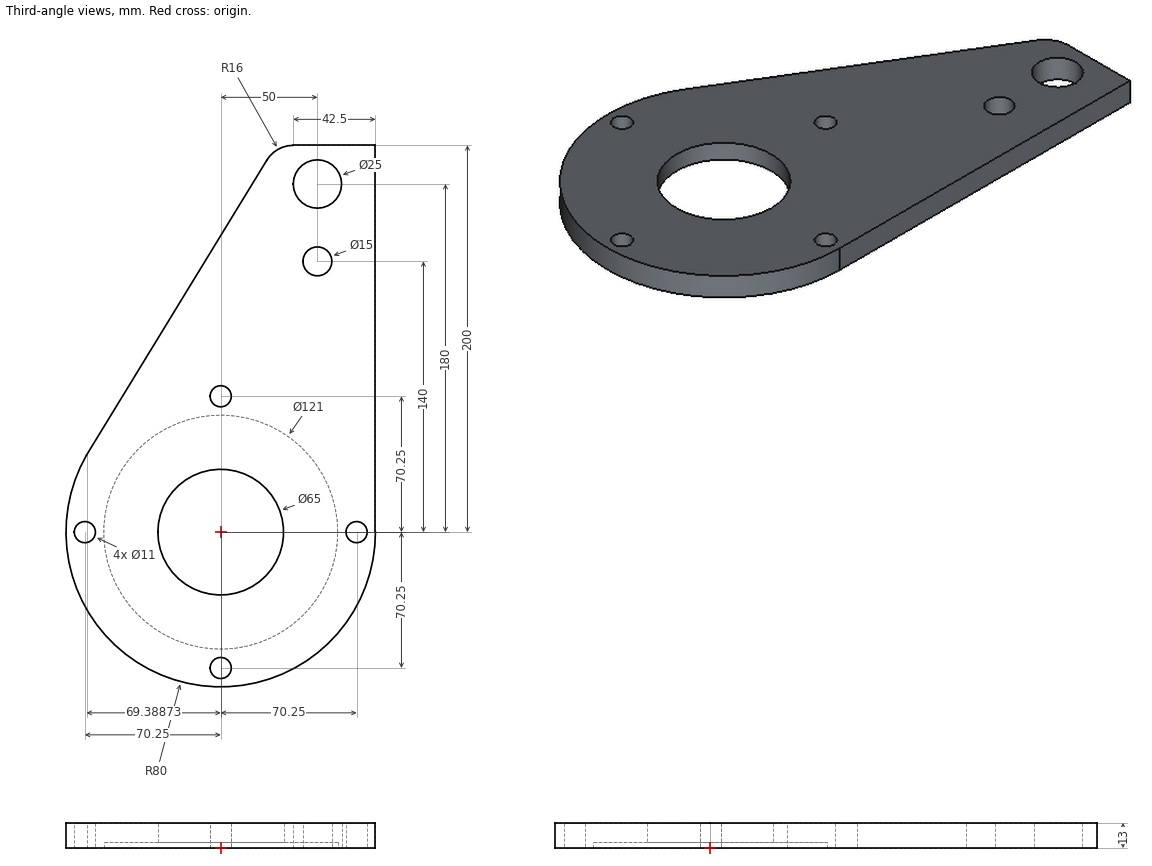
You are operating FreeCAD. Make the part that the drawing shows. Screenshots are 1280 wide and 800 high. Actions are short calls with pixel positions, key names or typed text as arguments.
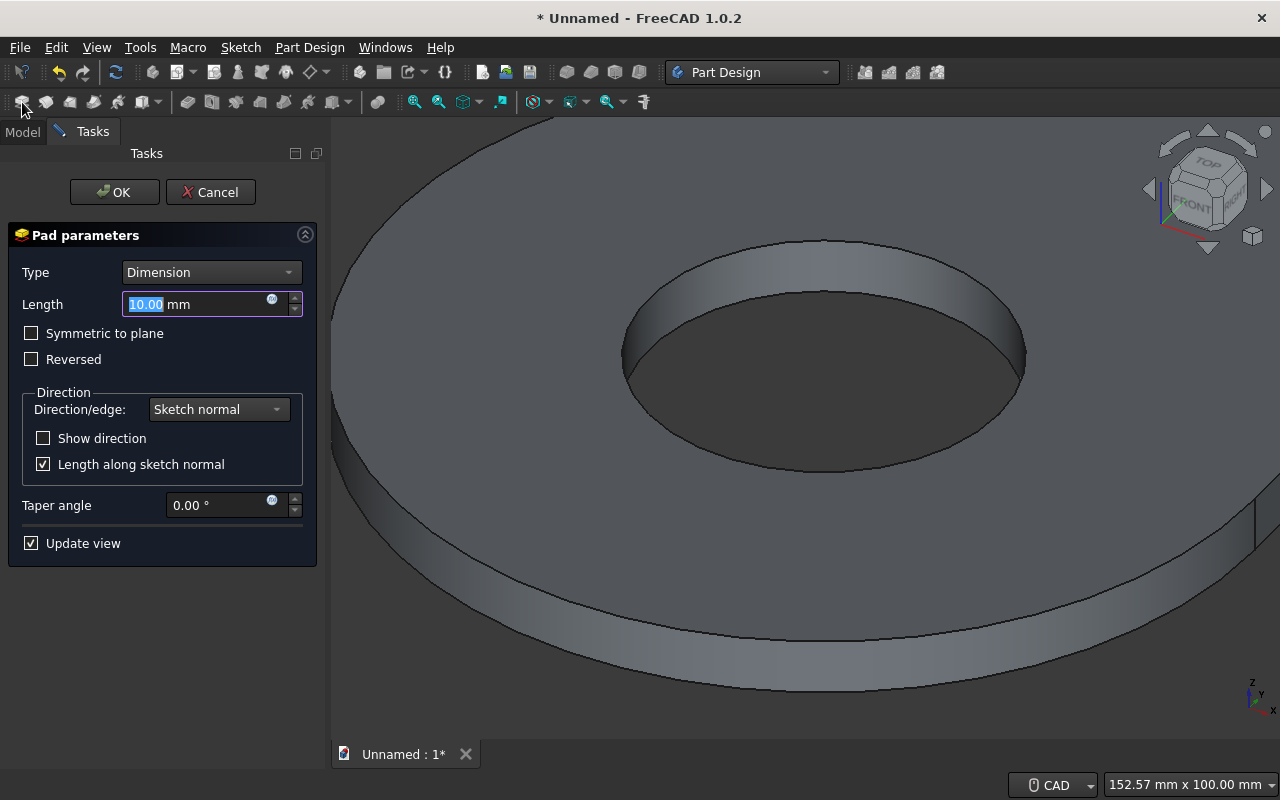
text(13)
key(Tab)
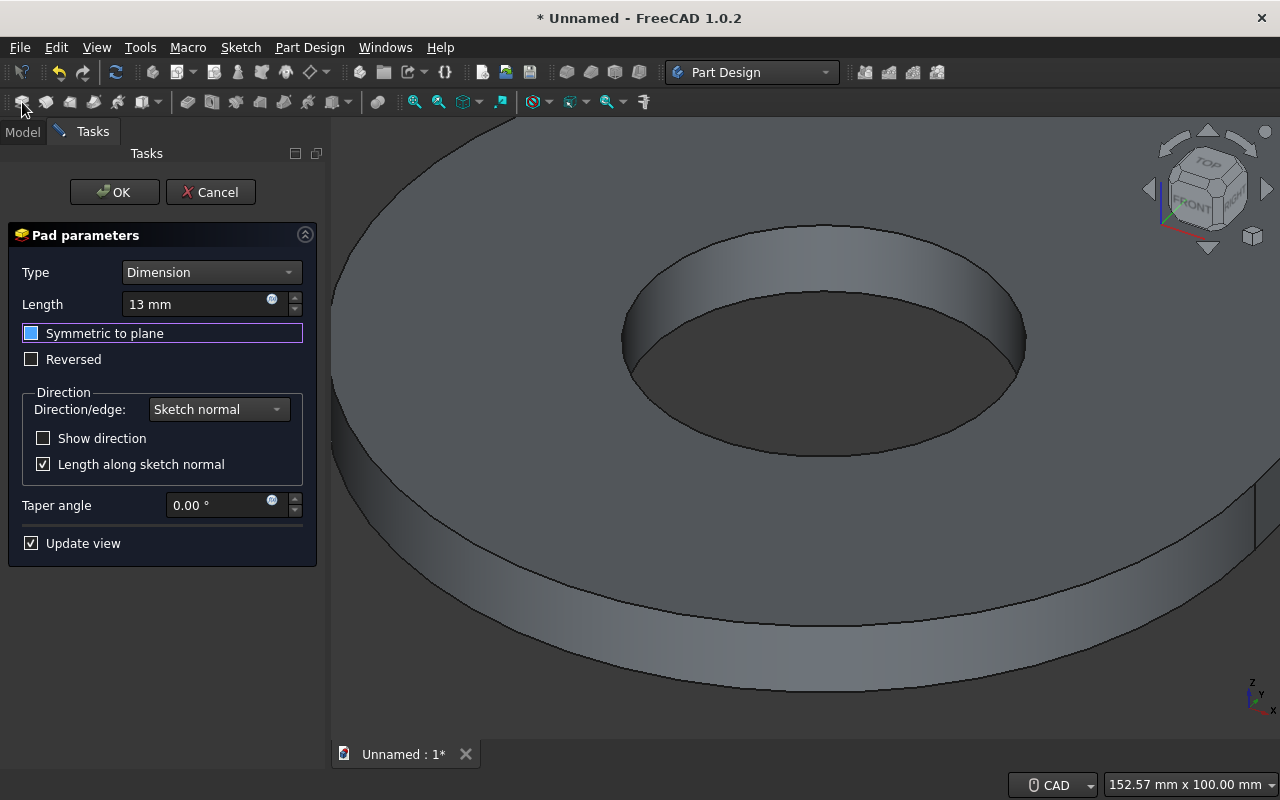
click(115, 192)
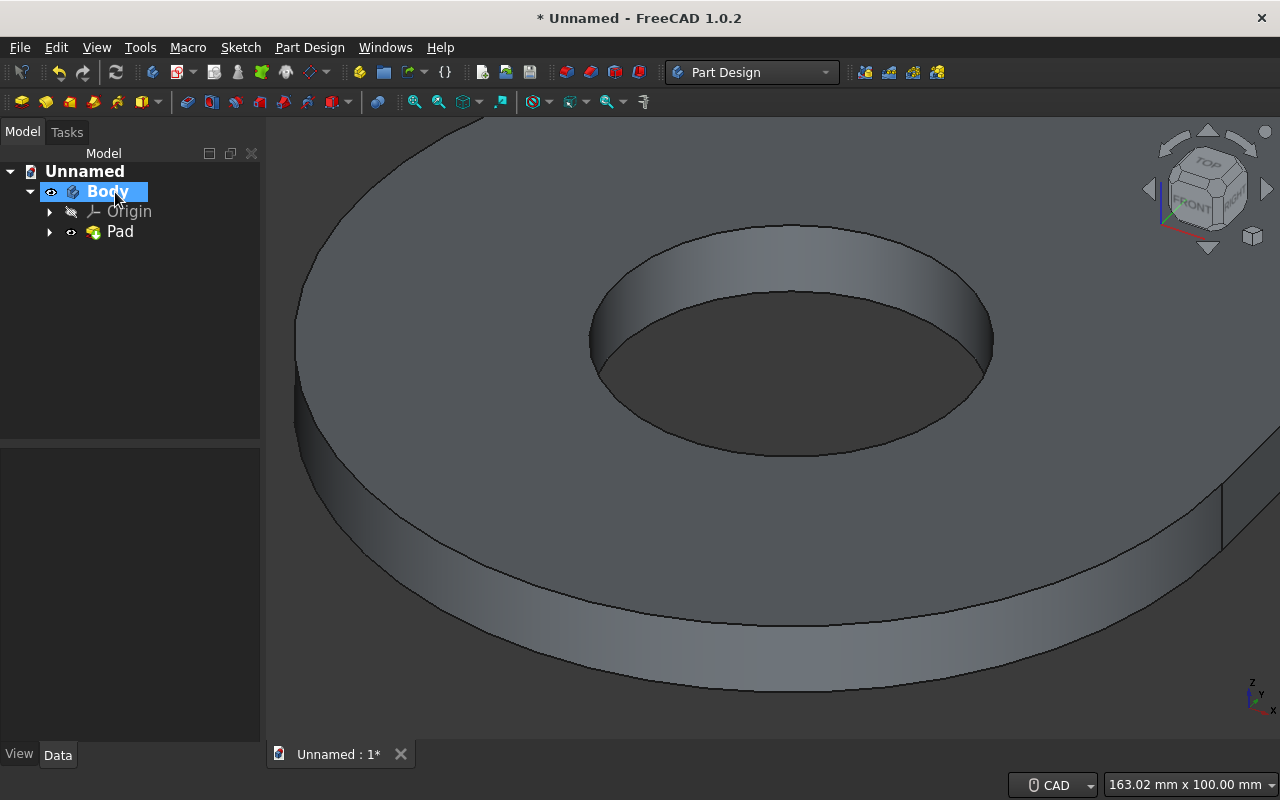
click(416, 102)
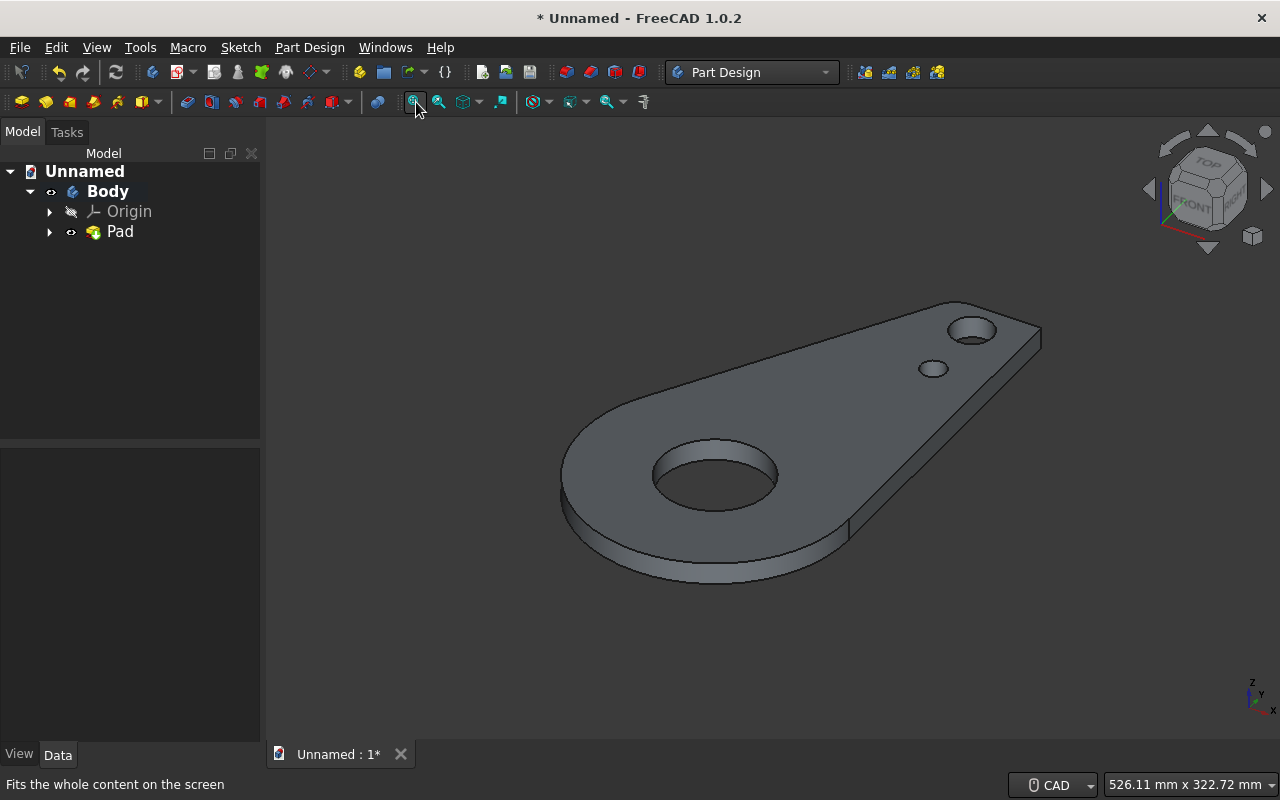
click(50, 212)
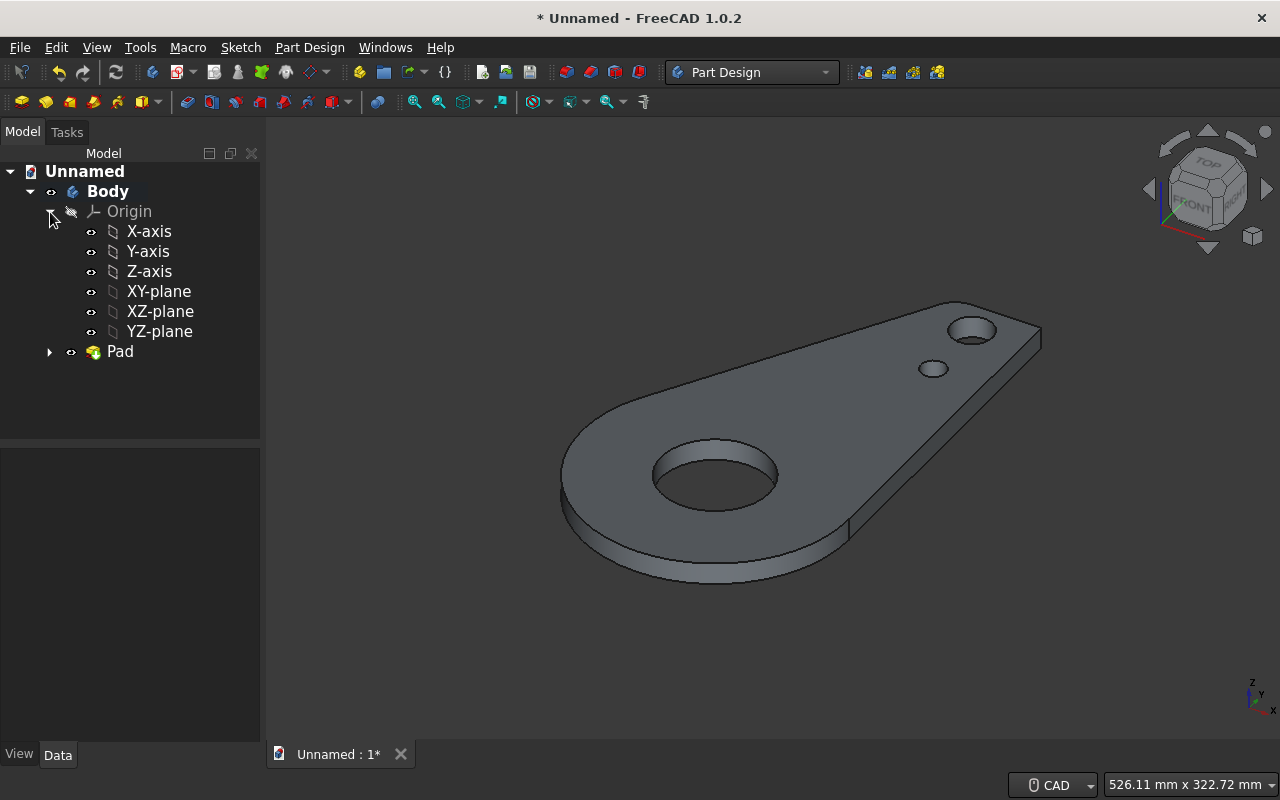
click(136, 292)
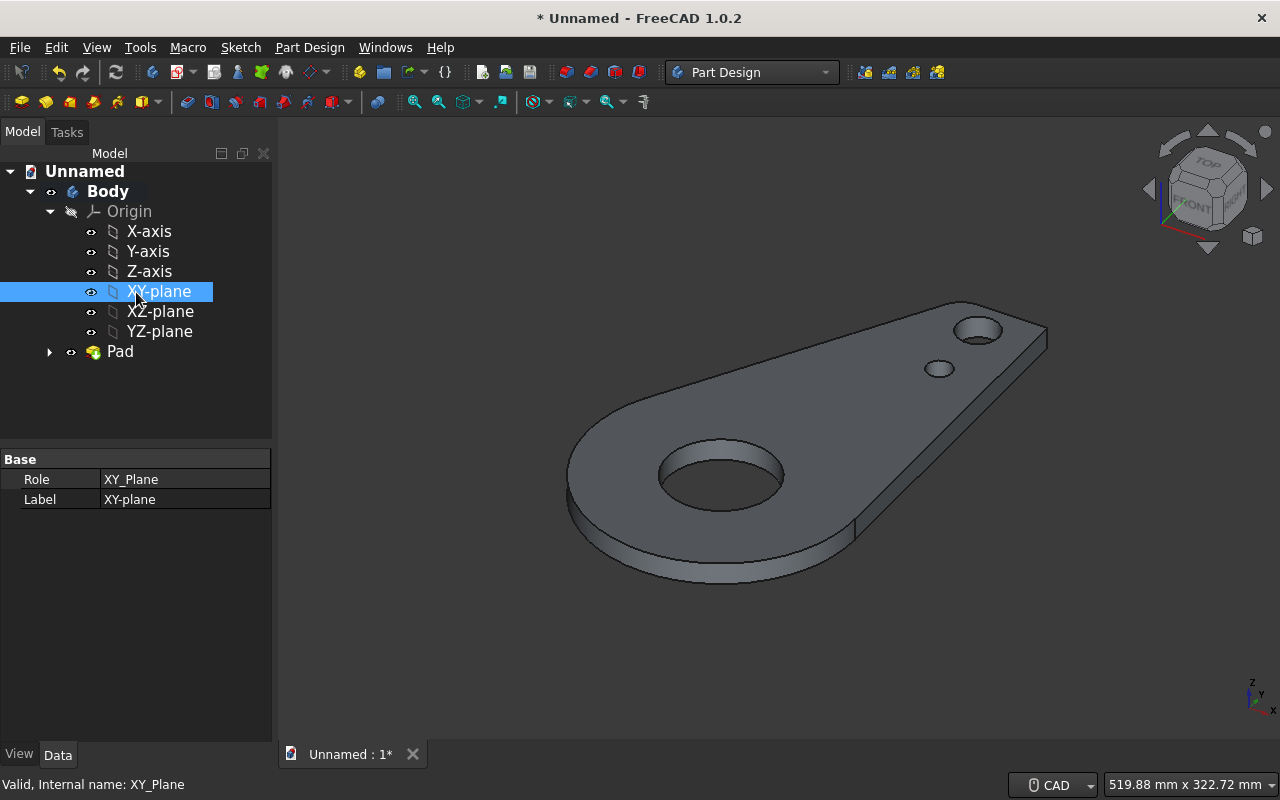
click(310, 72)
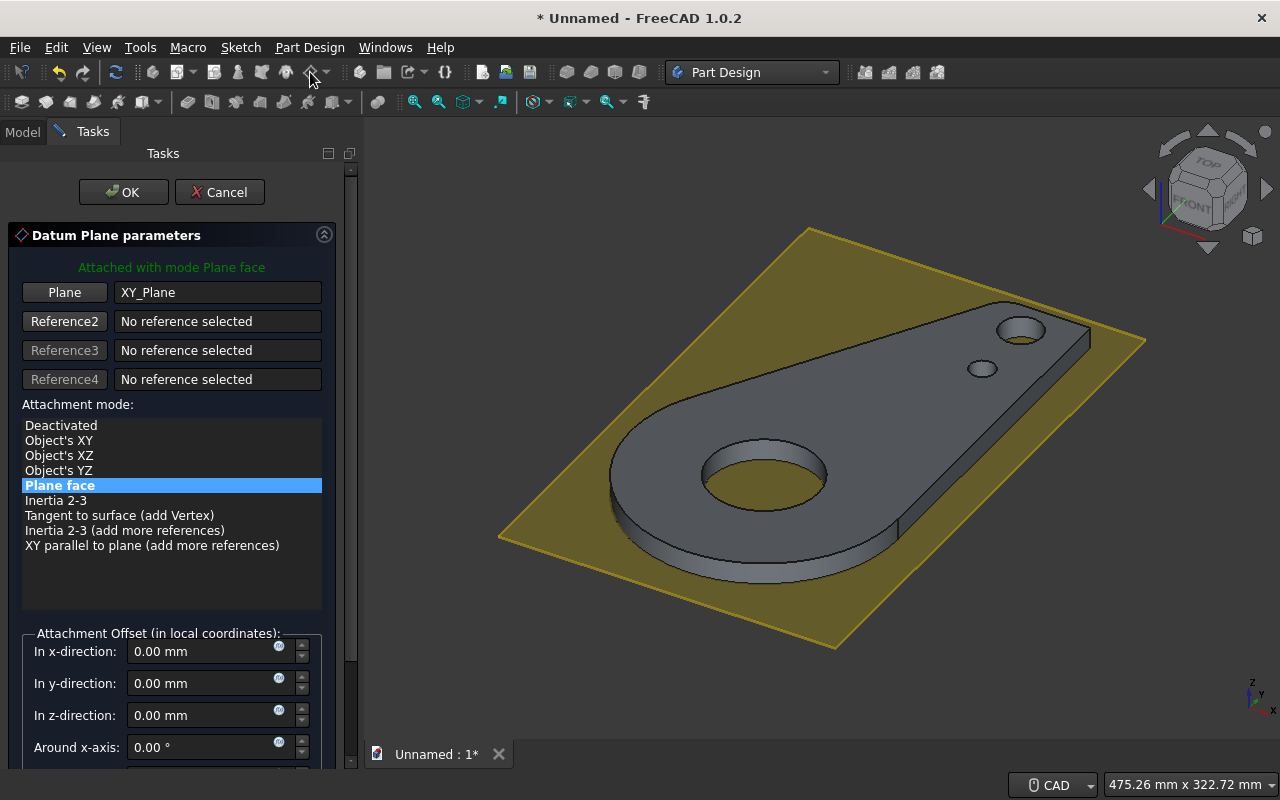
triple_click(210, 715)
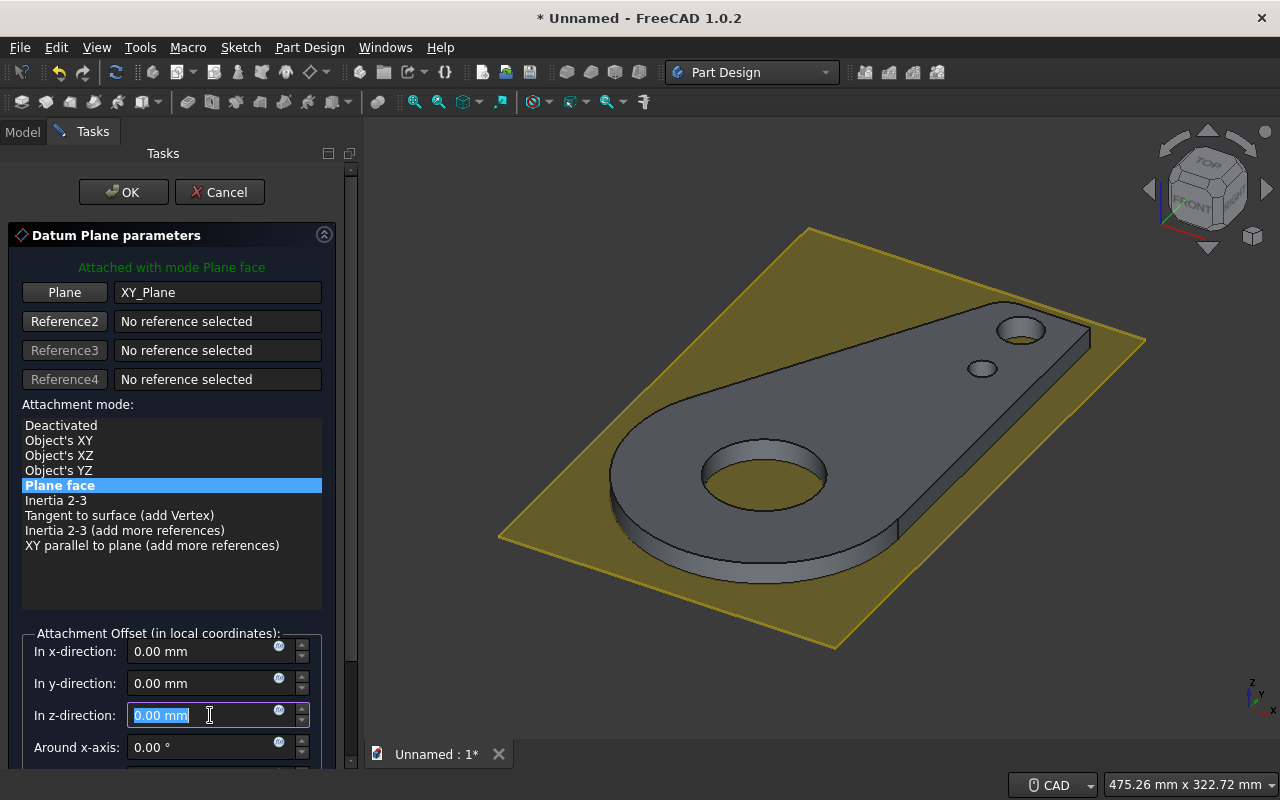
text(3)
key(Tab)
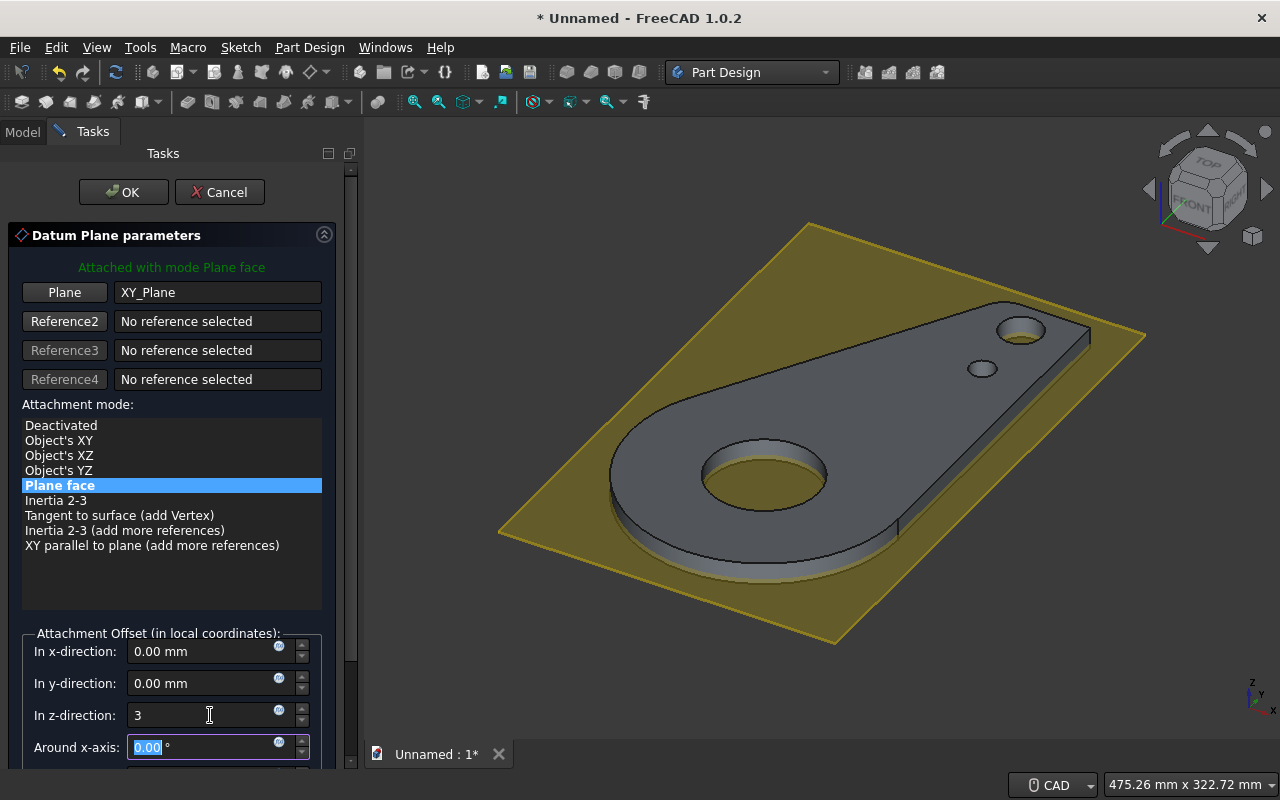
click(124, 192)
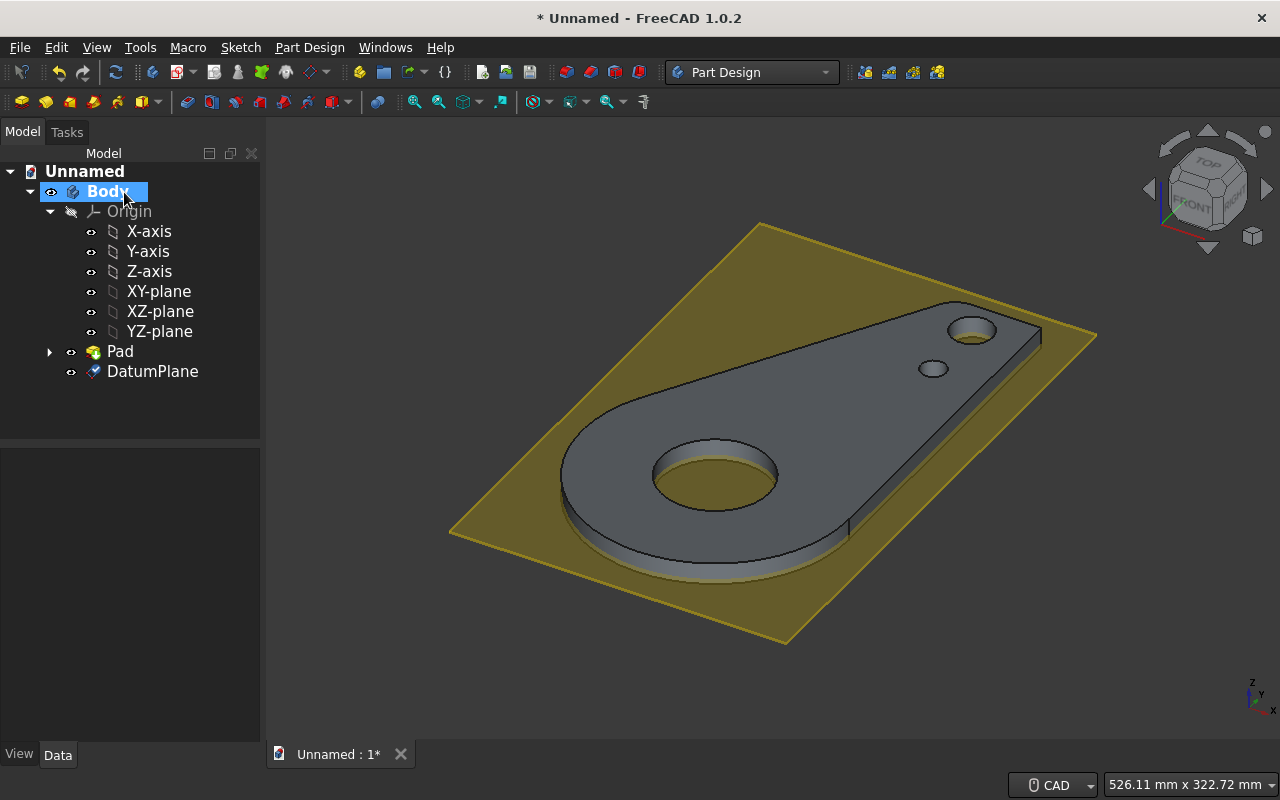
click(116, 372)